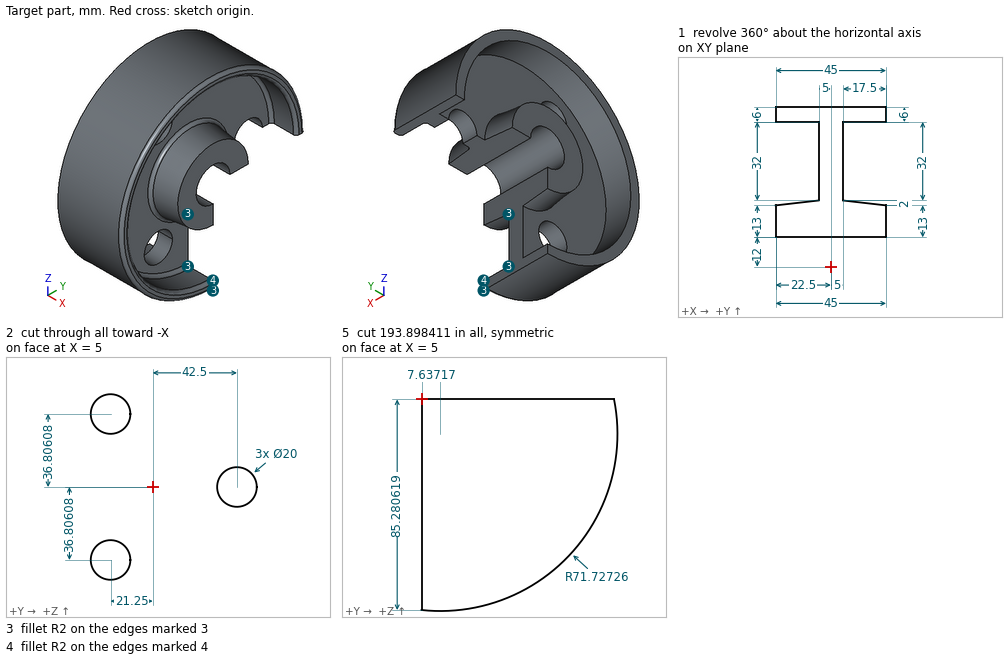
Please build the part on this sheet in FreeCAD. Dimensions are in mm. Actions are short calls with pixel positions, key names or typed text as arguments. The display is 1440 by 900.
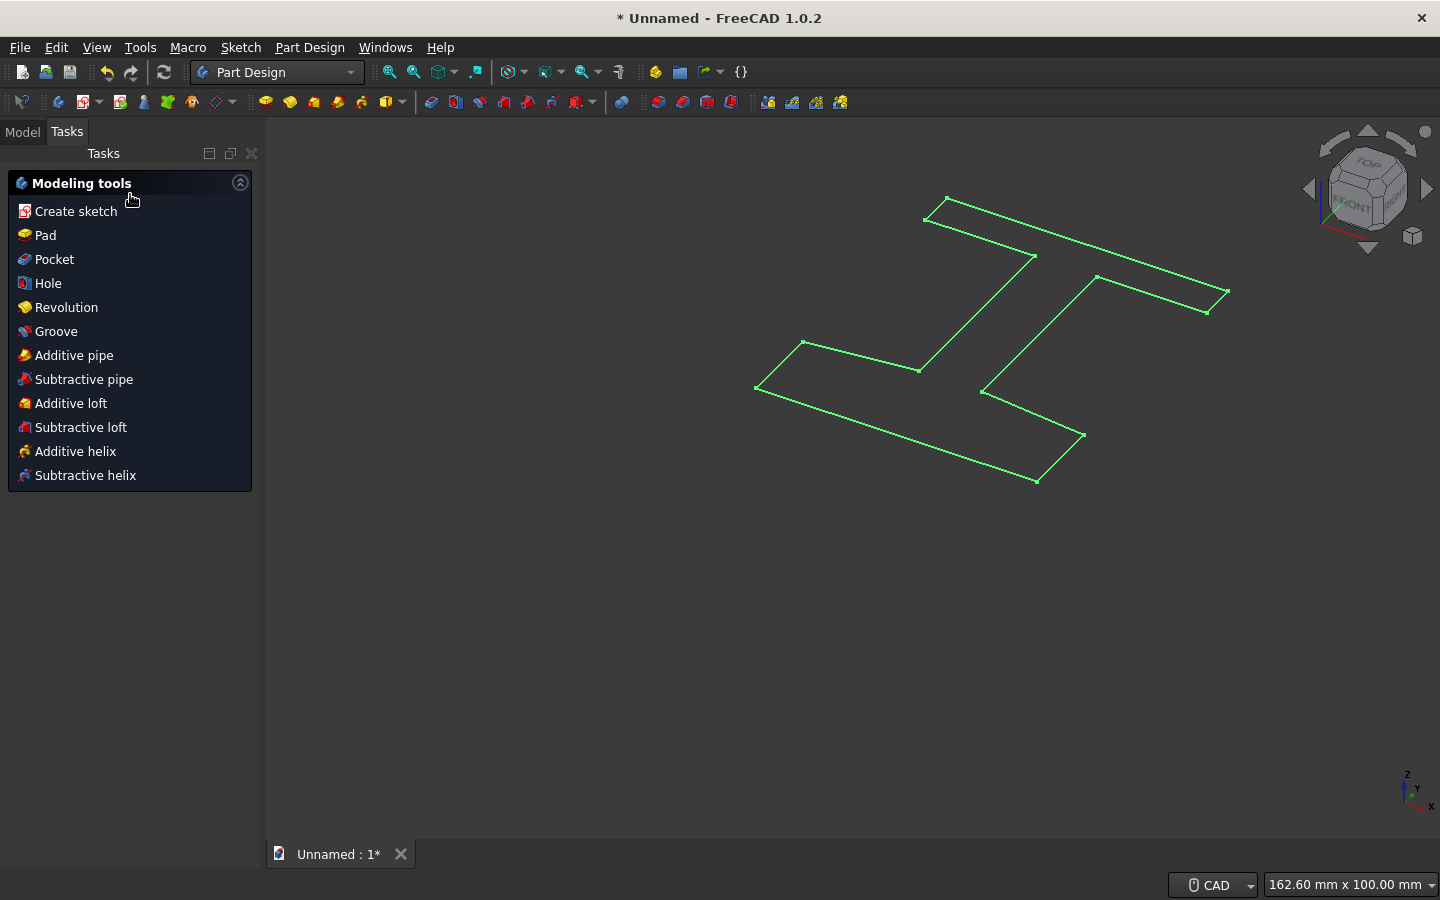
click(290, 102)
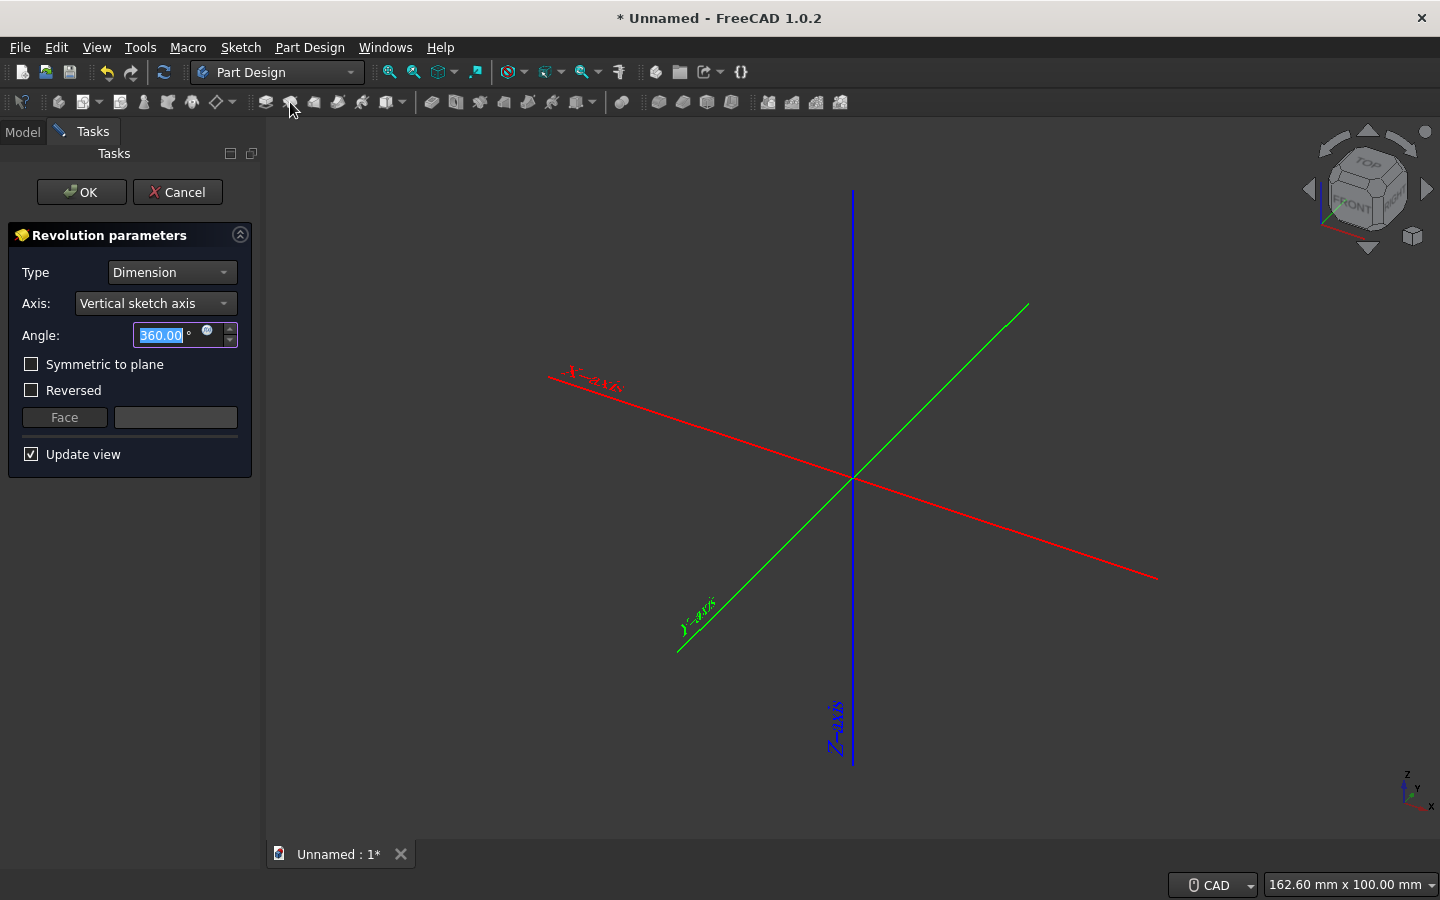
click(156, 304)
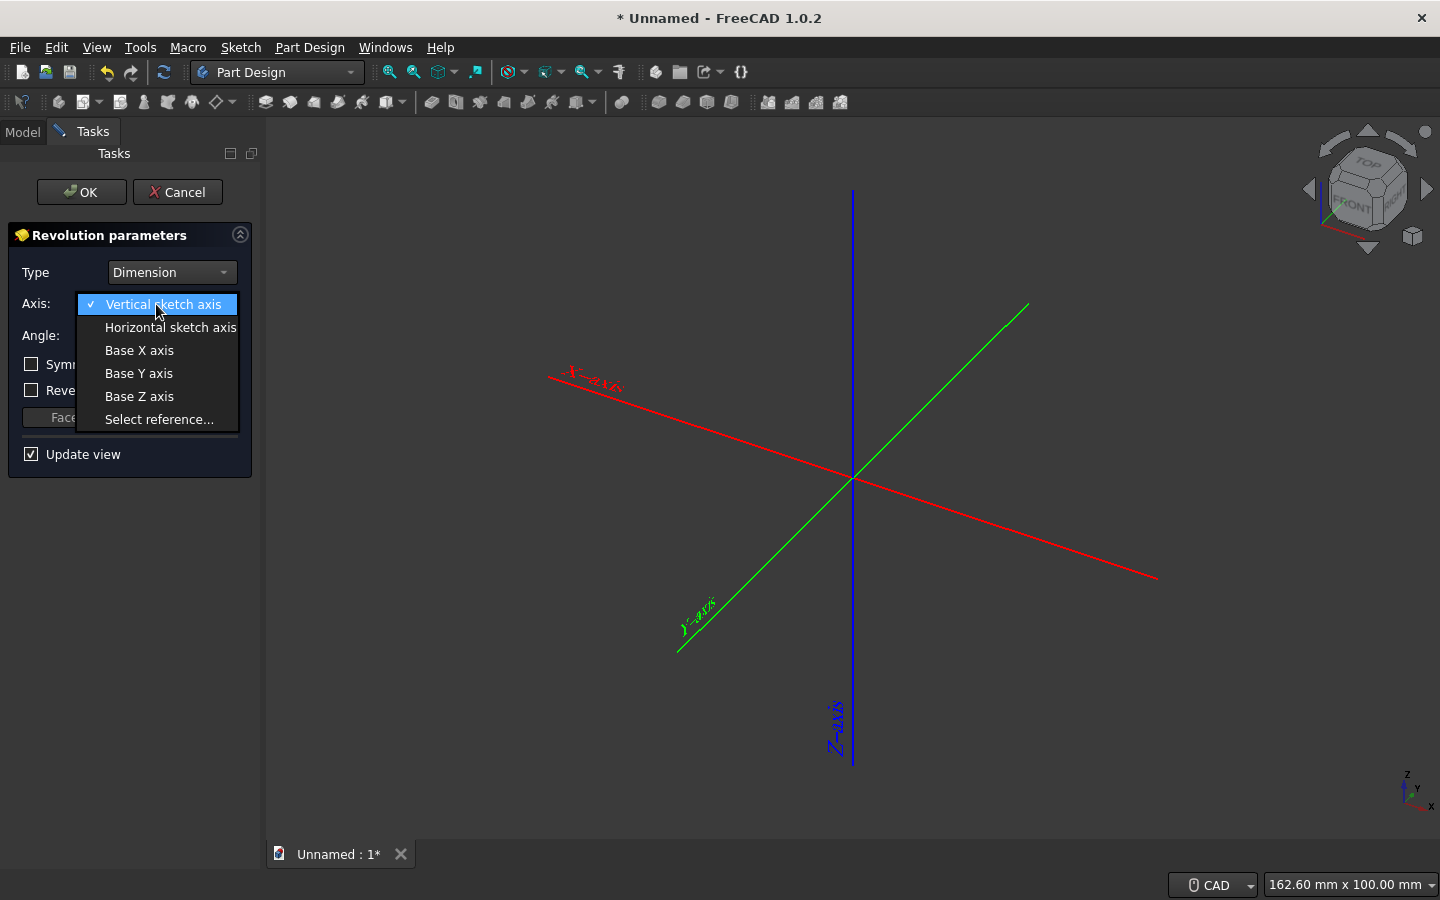
click(156, 328)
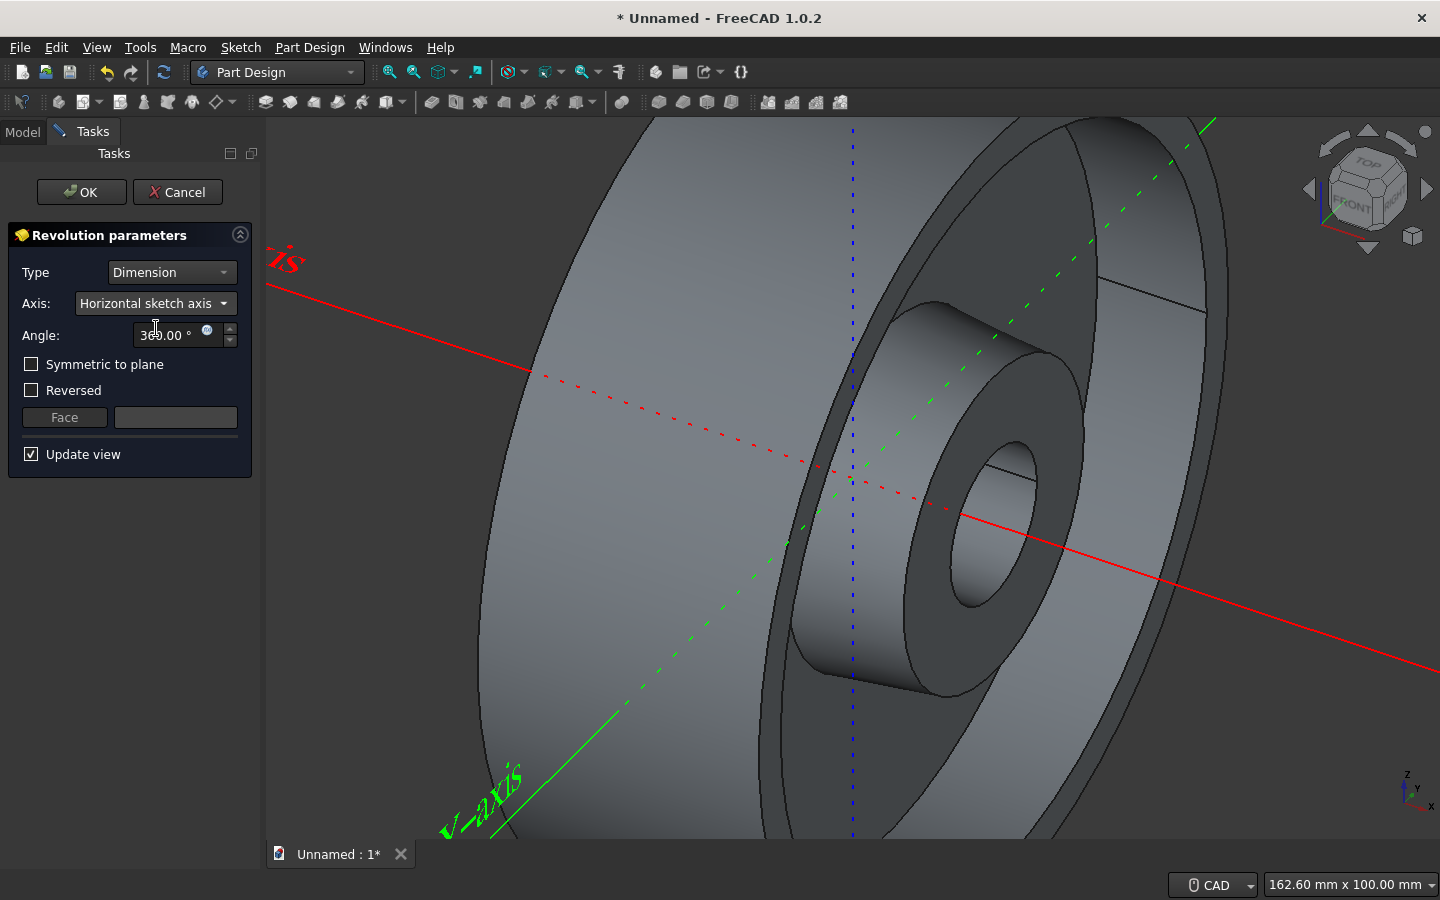
click(82, 192)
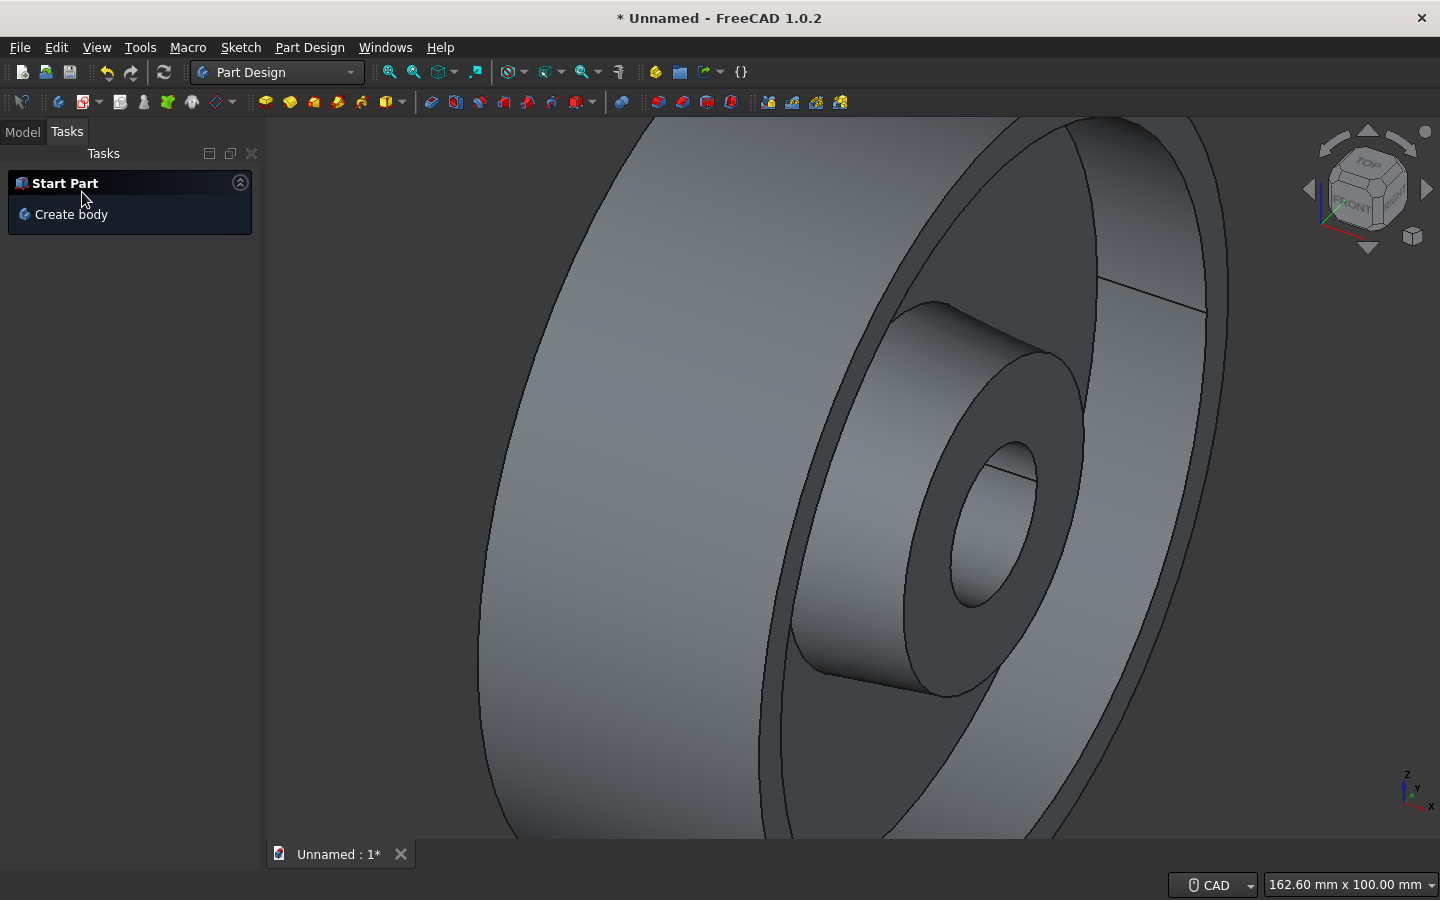
key(v)
key(f)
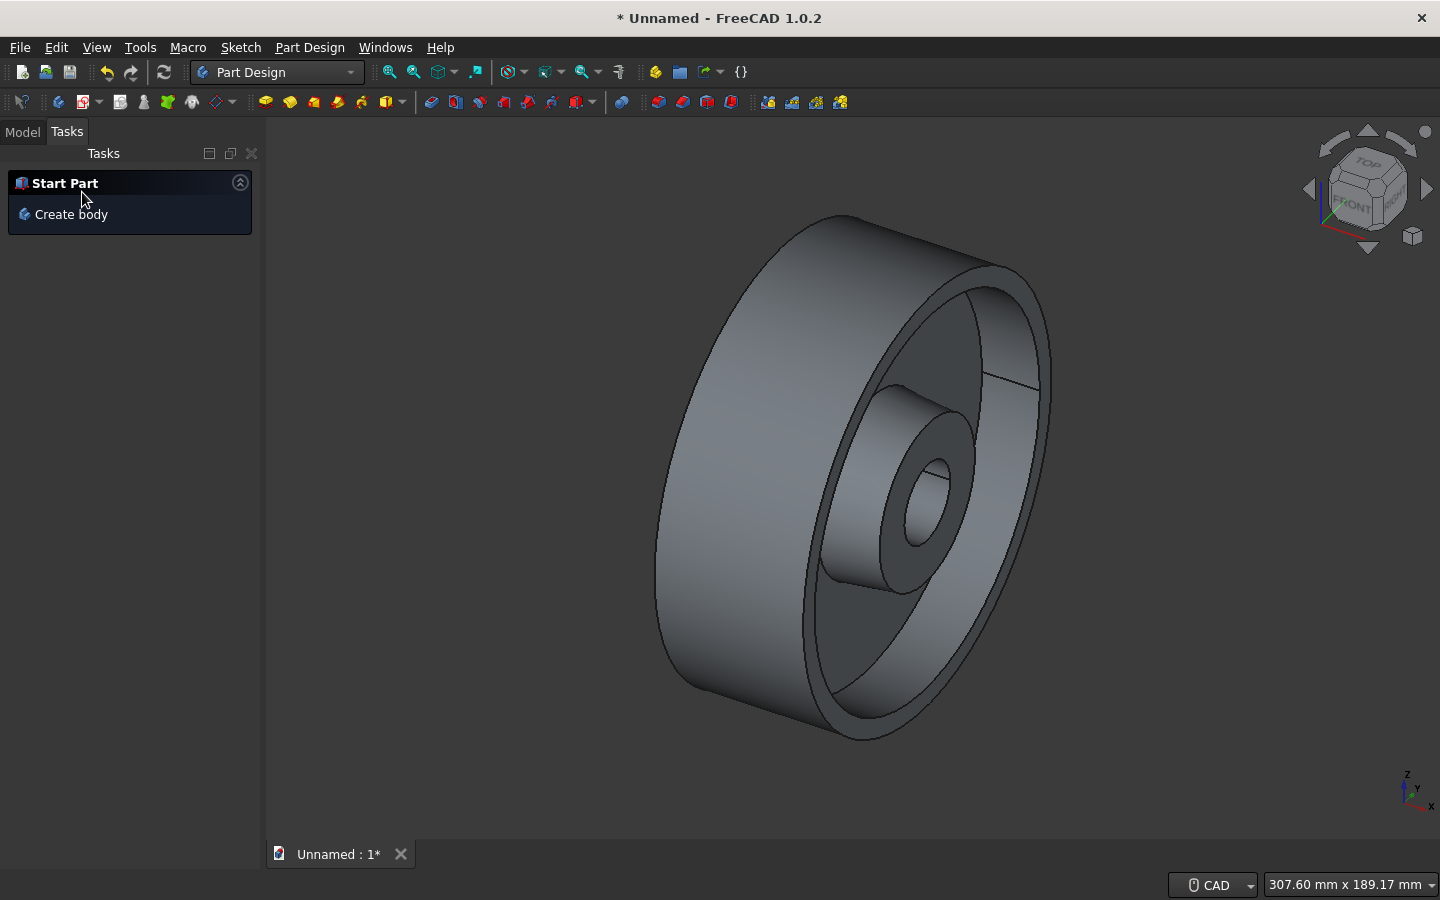
click(837, 620)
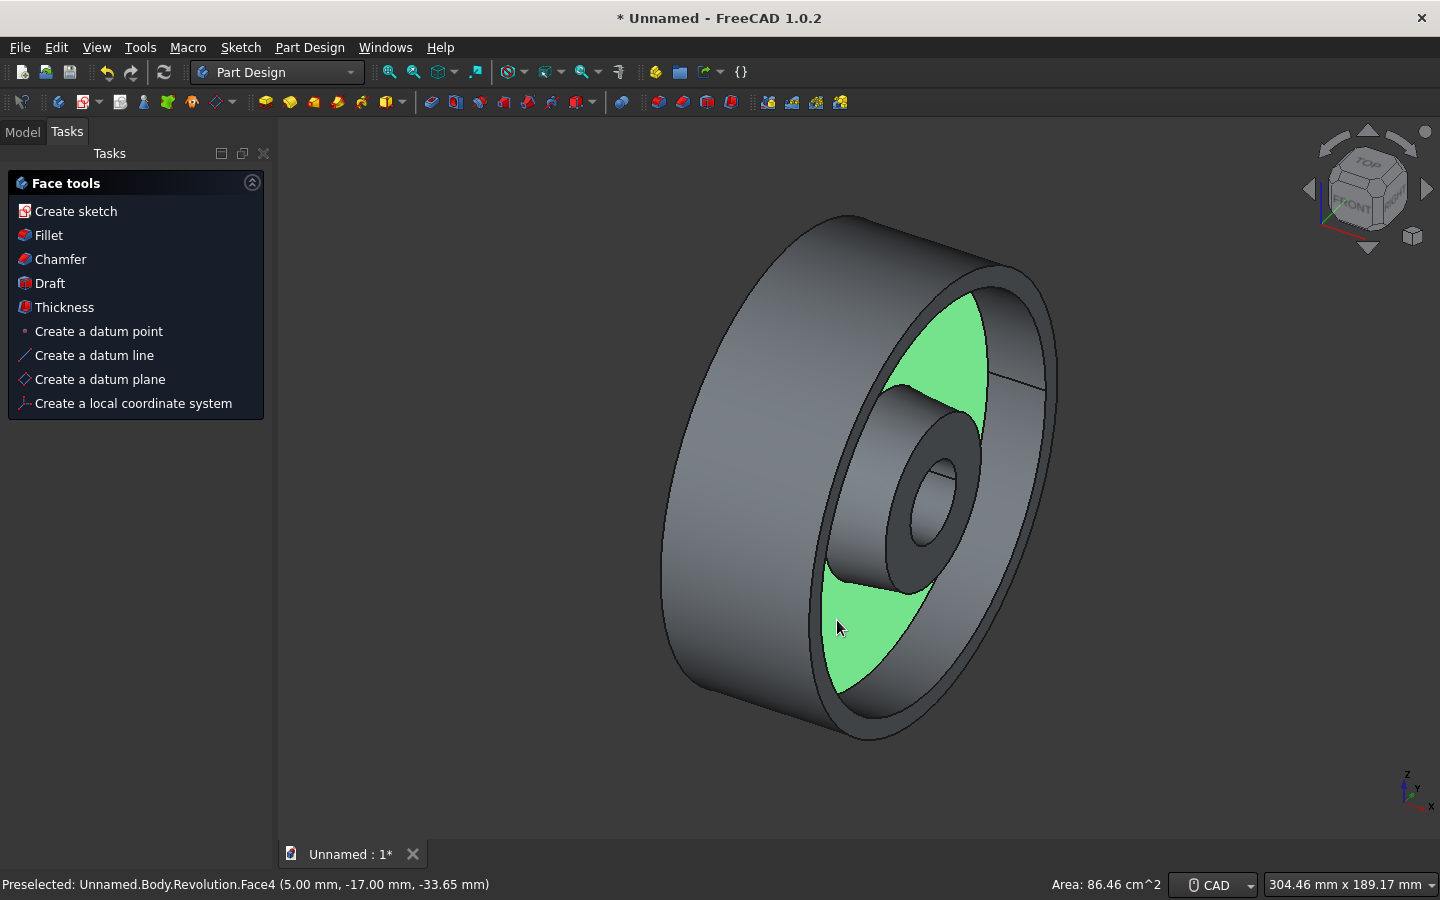
click(84, 102)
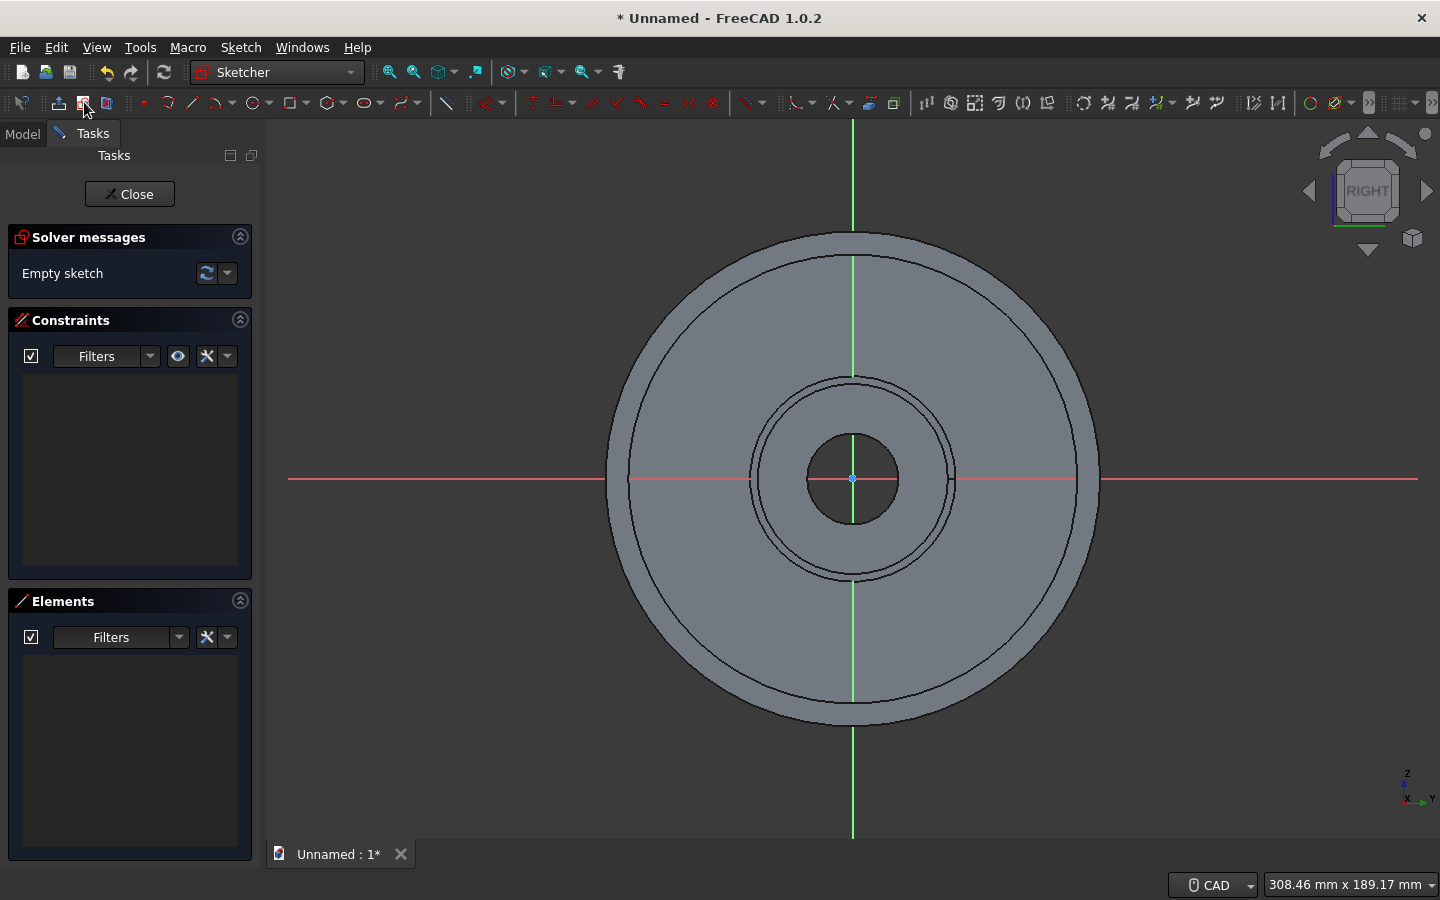
click(254, 104)